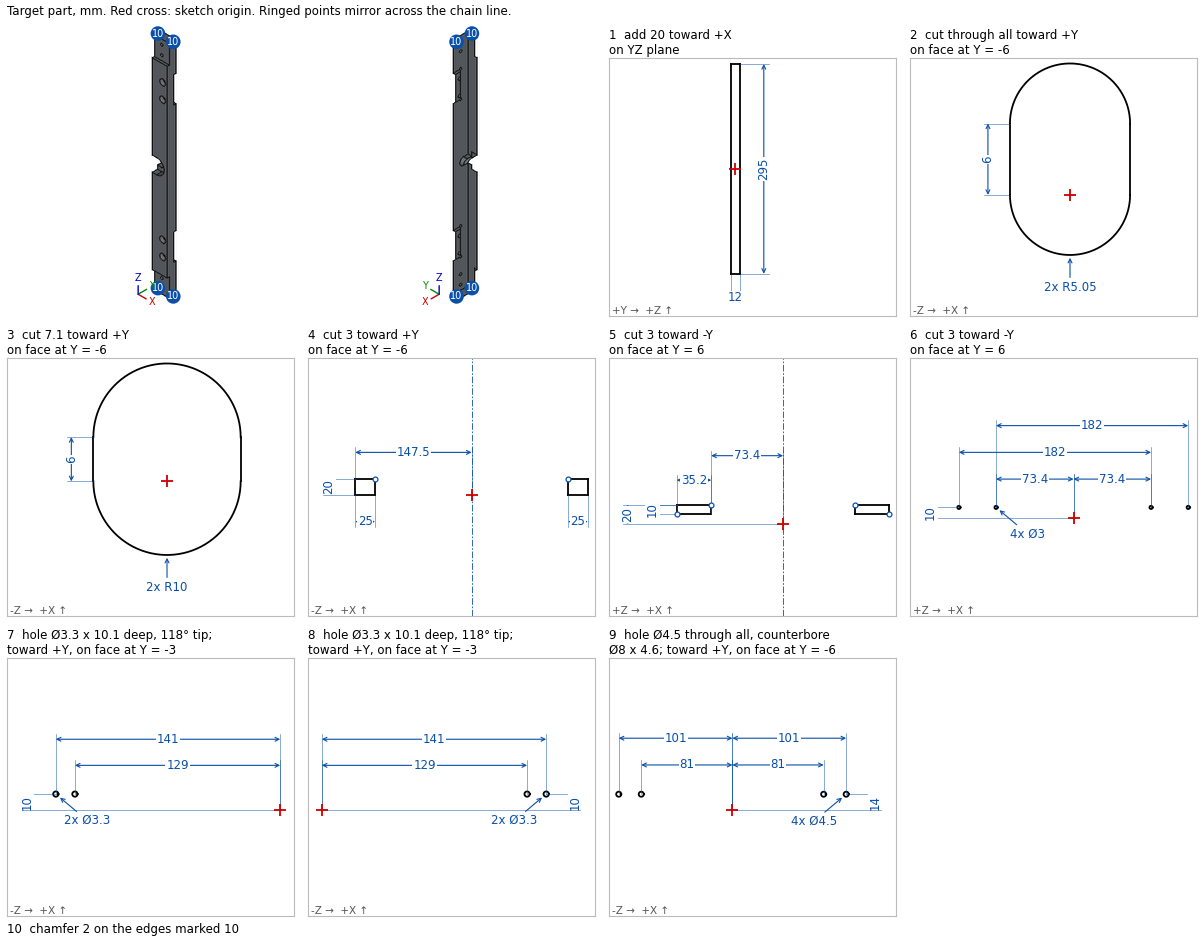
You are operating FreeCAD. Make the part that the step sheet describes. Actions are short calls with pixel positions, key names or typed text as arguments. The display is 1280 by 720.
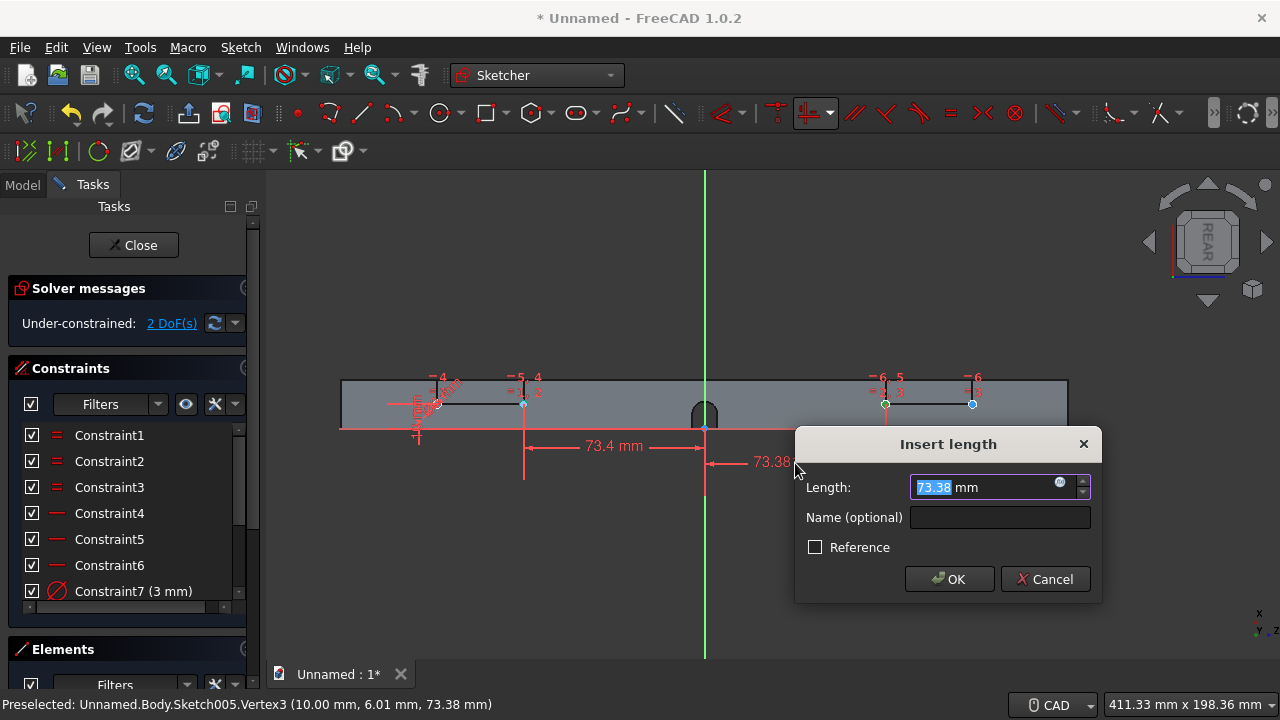
text(73.4)
key(Return)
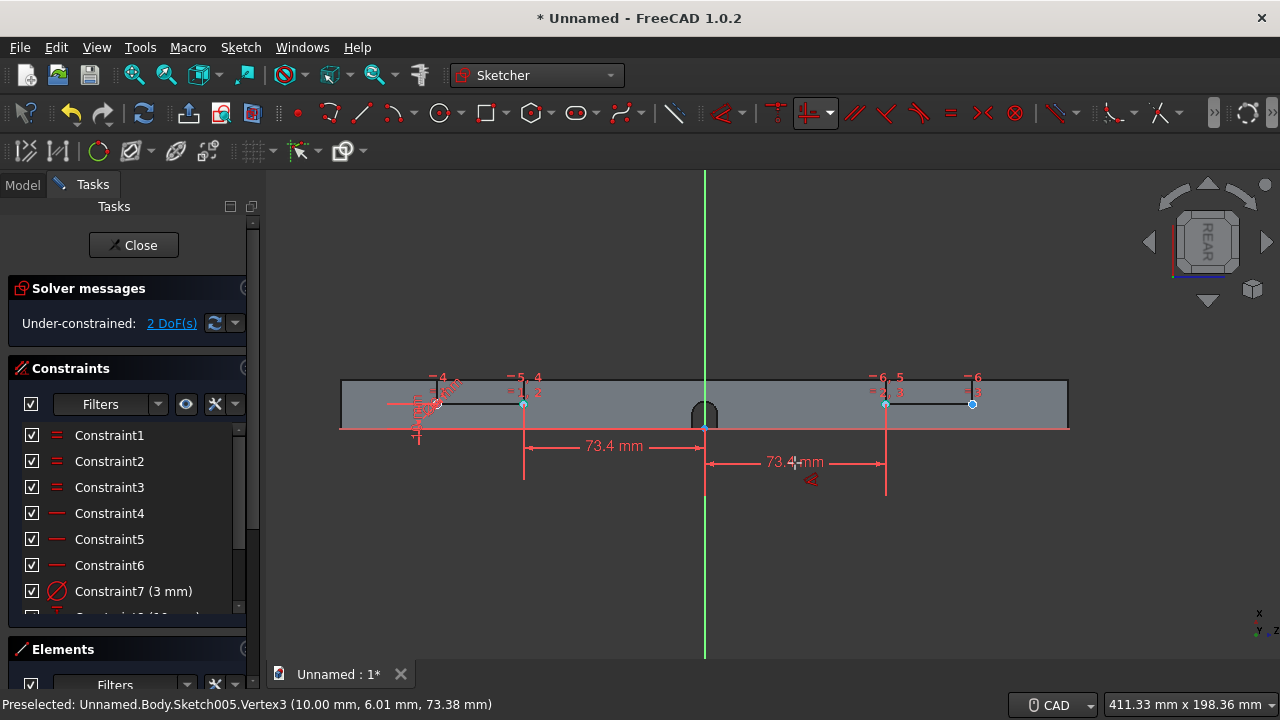
click(437, 404)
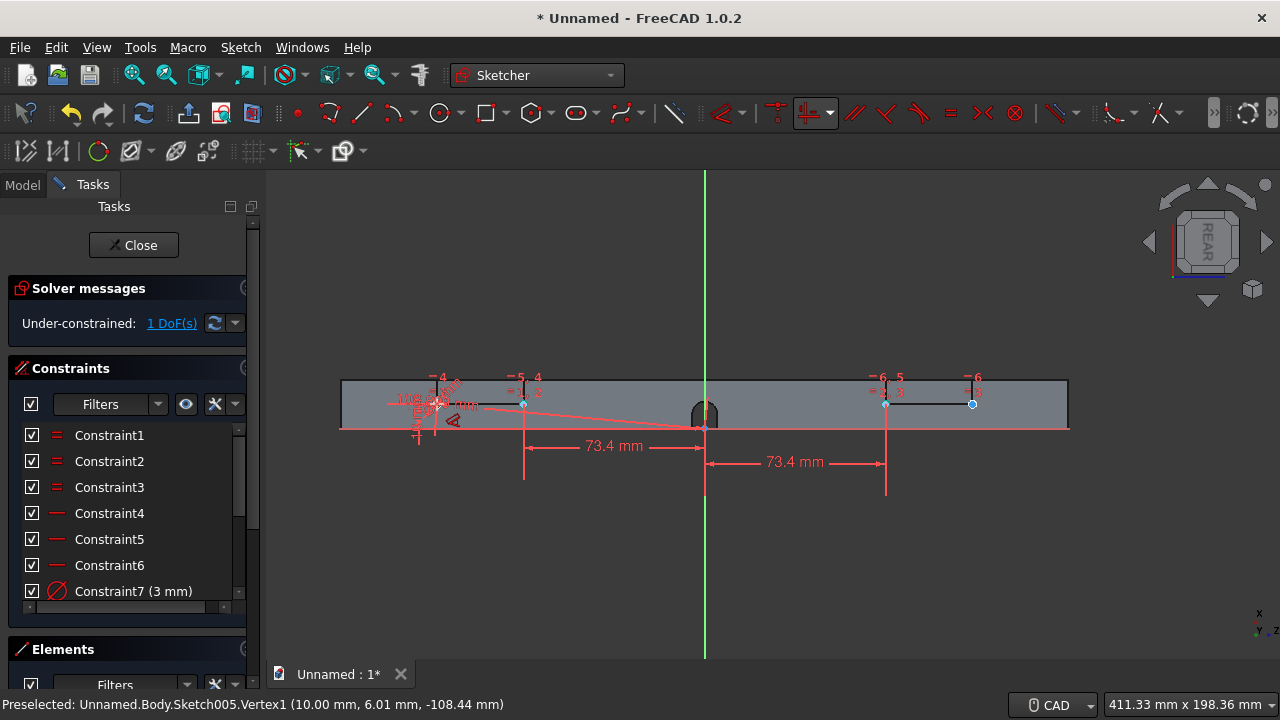
click(886, 404)
click(662, 370)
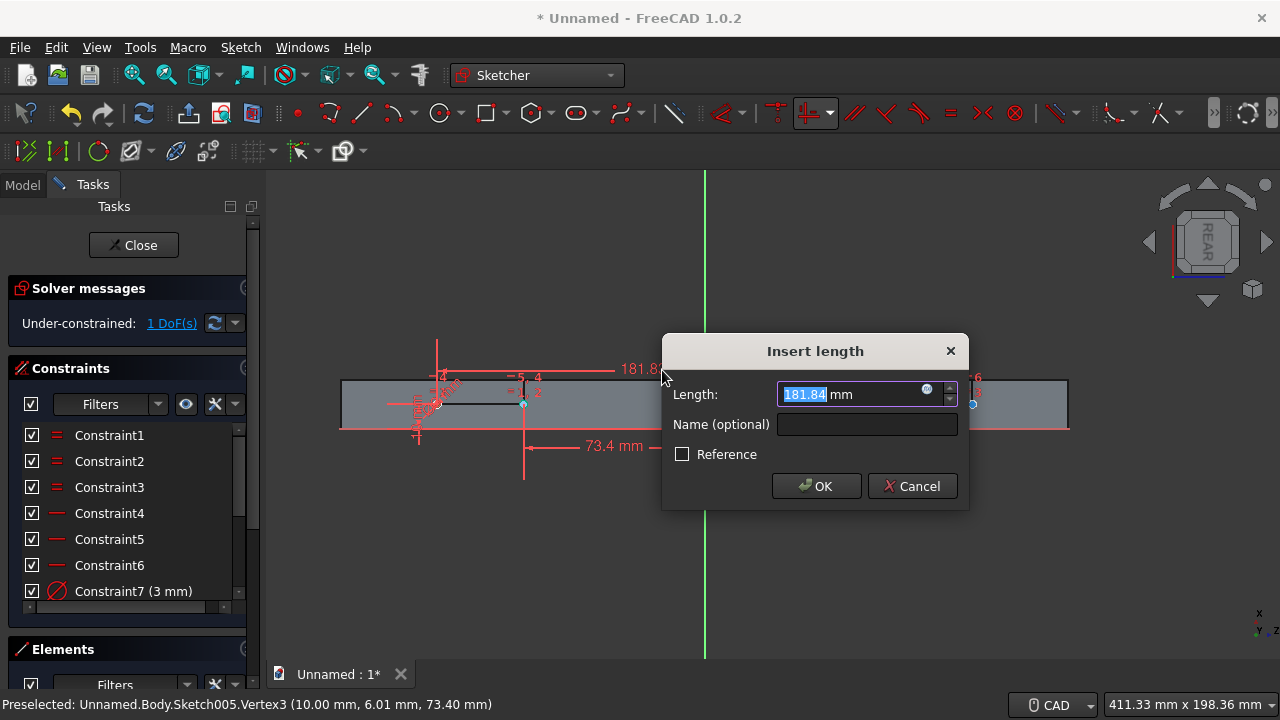
text(182)
key(Return)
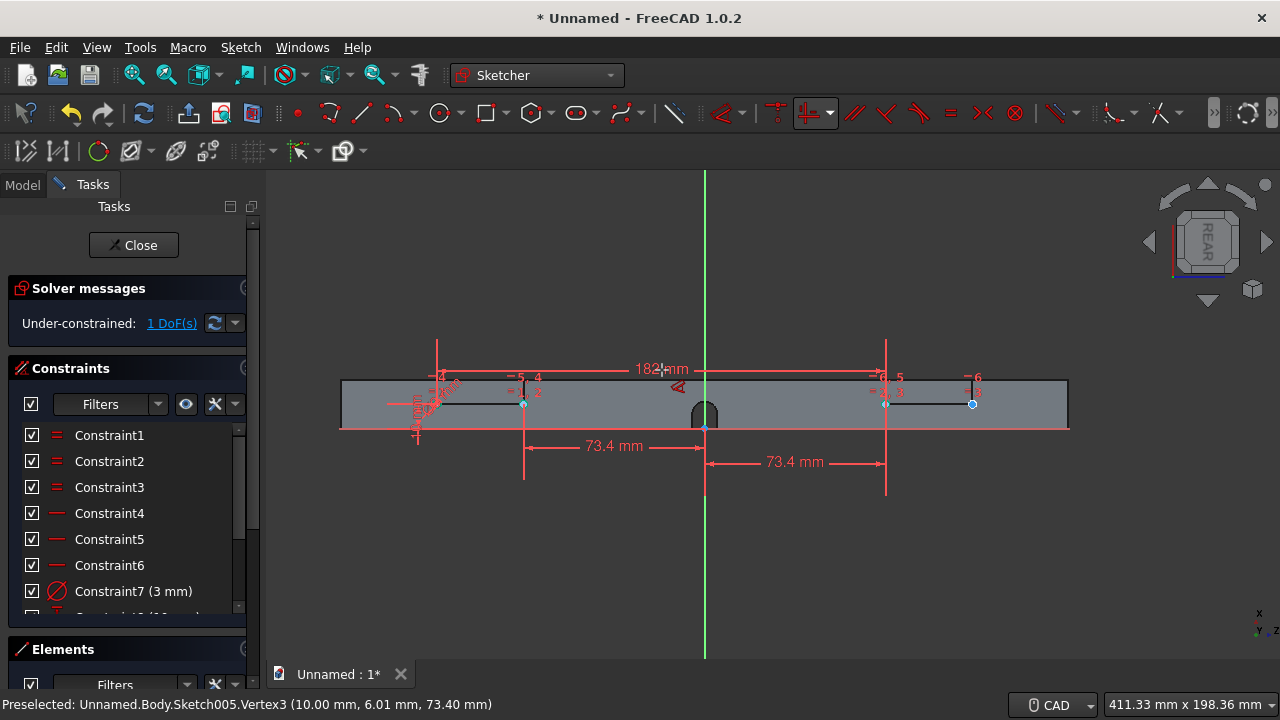
click(524, 404)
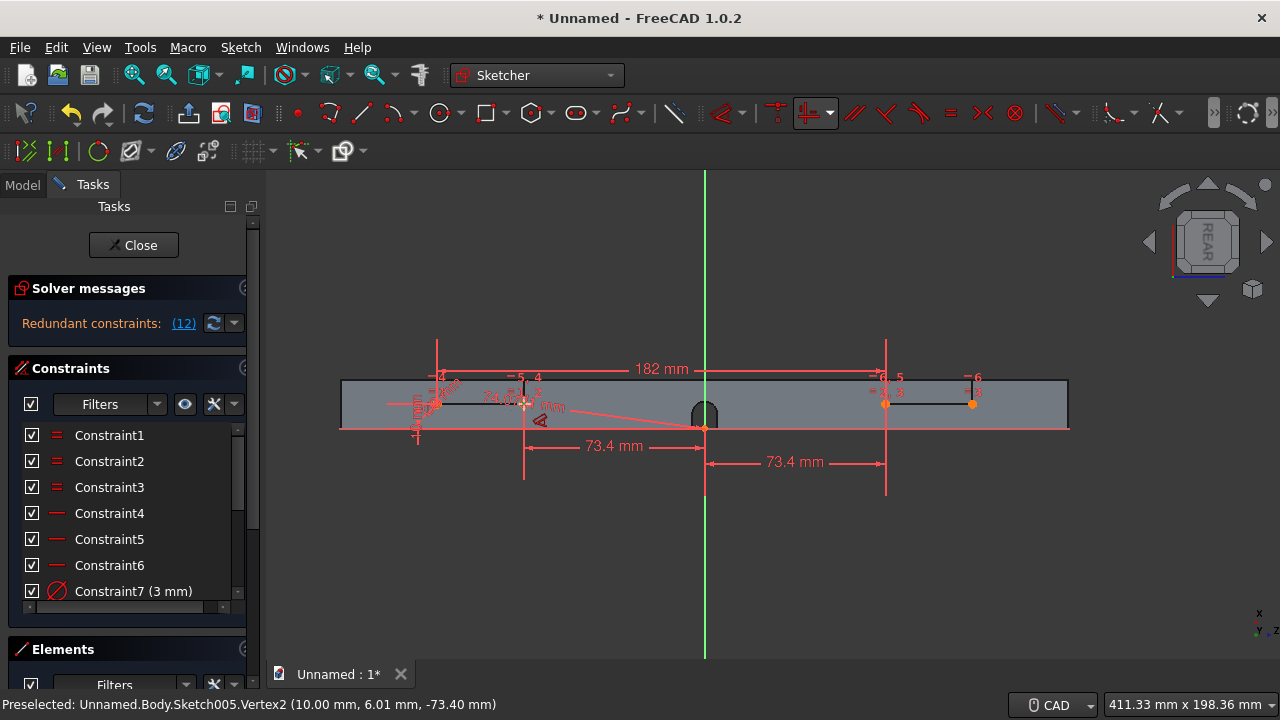
click(973, 404)
click(748, 370)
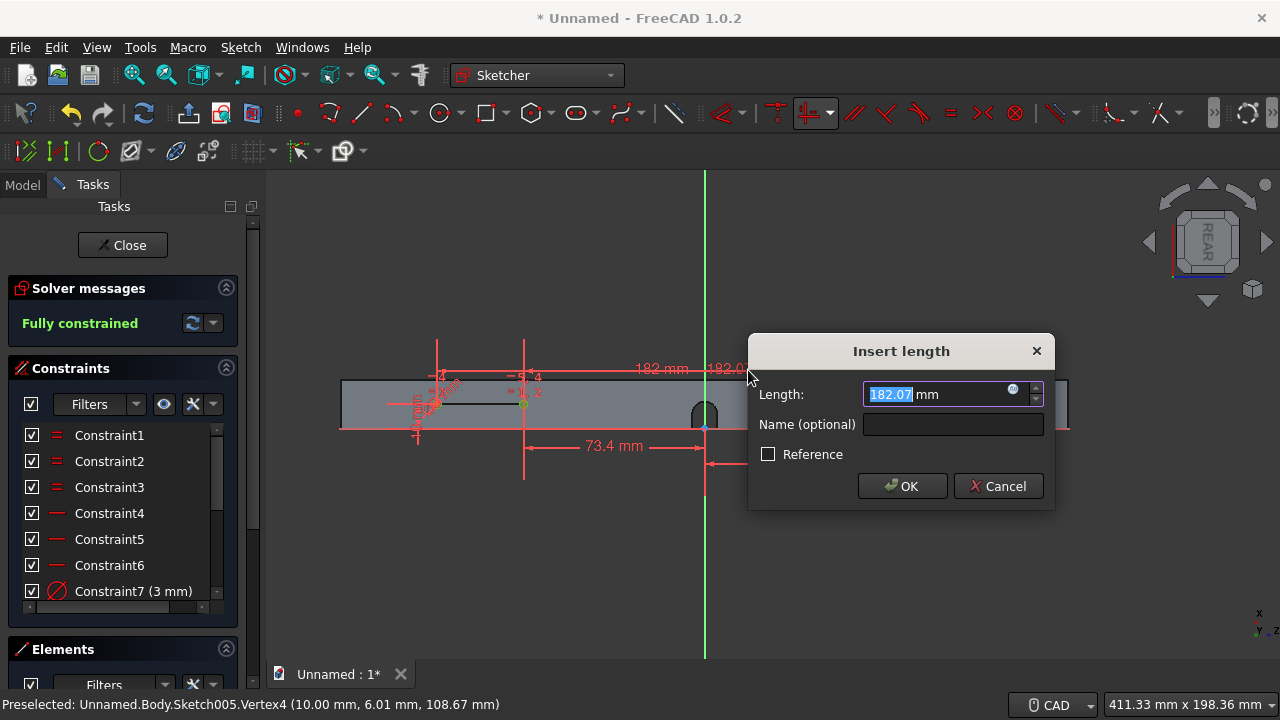
text(182)
key(Return)
key(Escape)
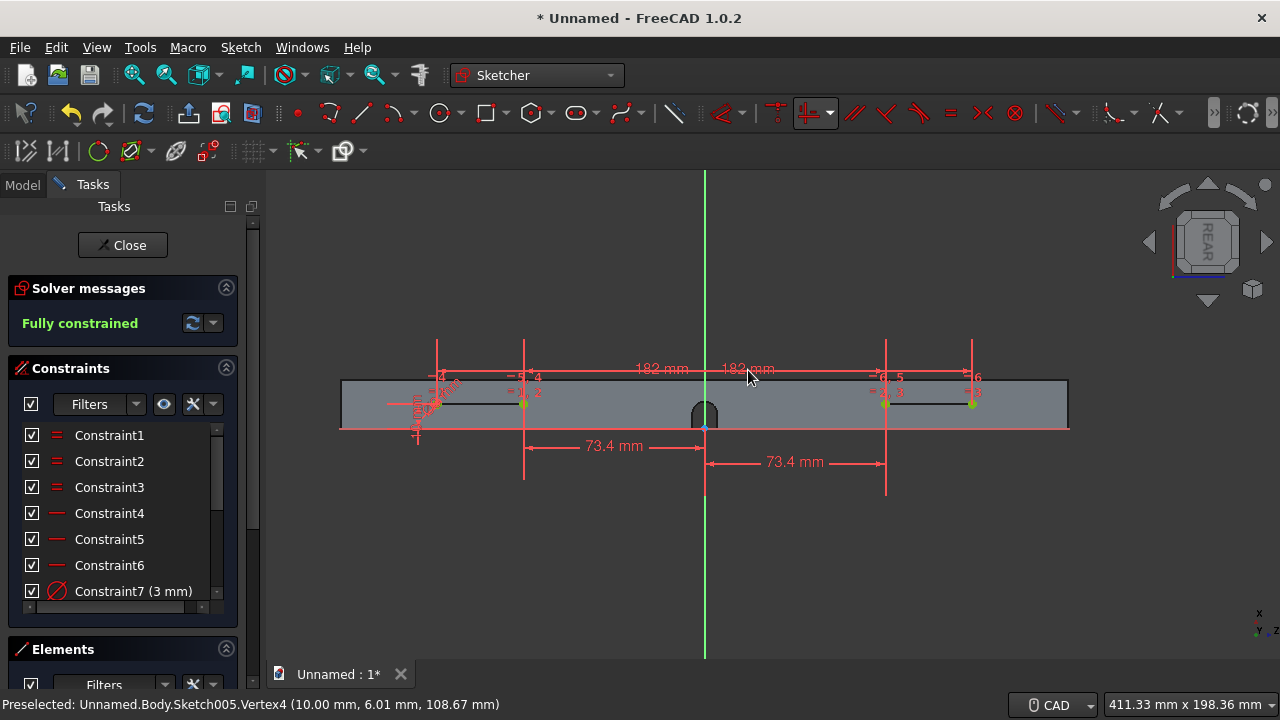
click(123, 245)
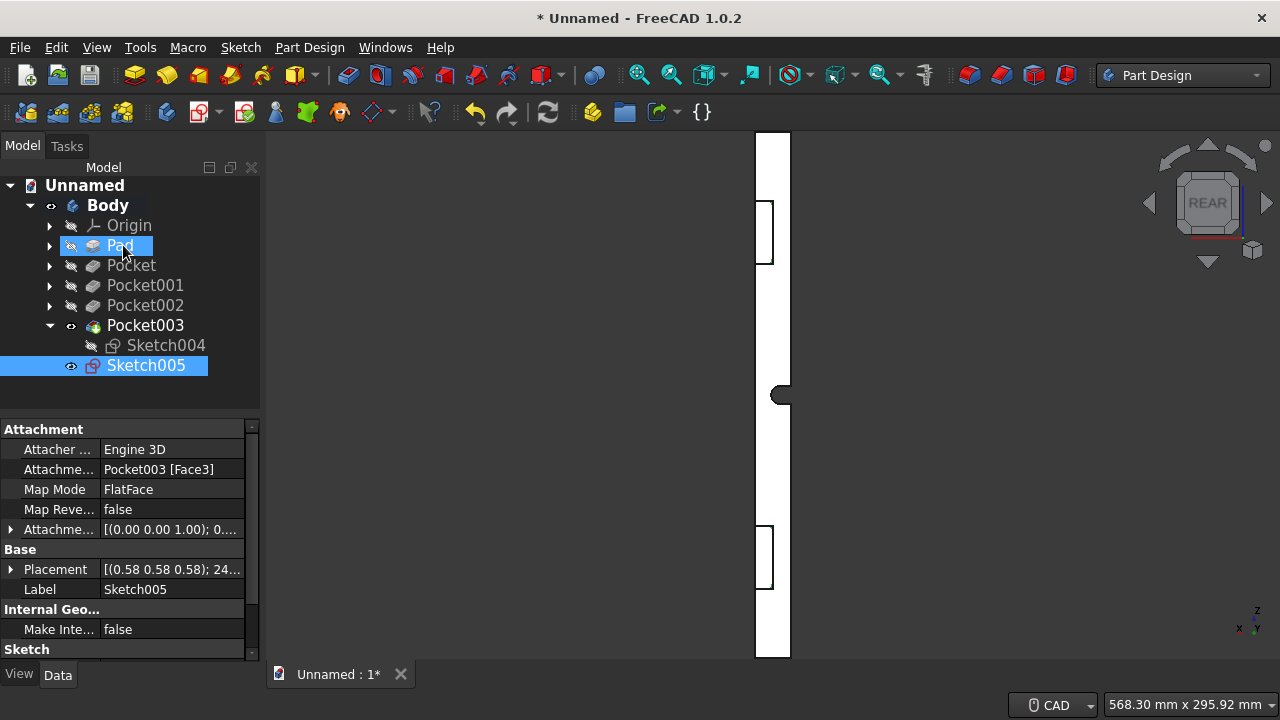
click(350, 76)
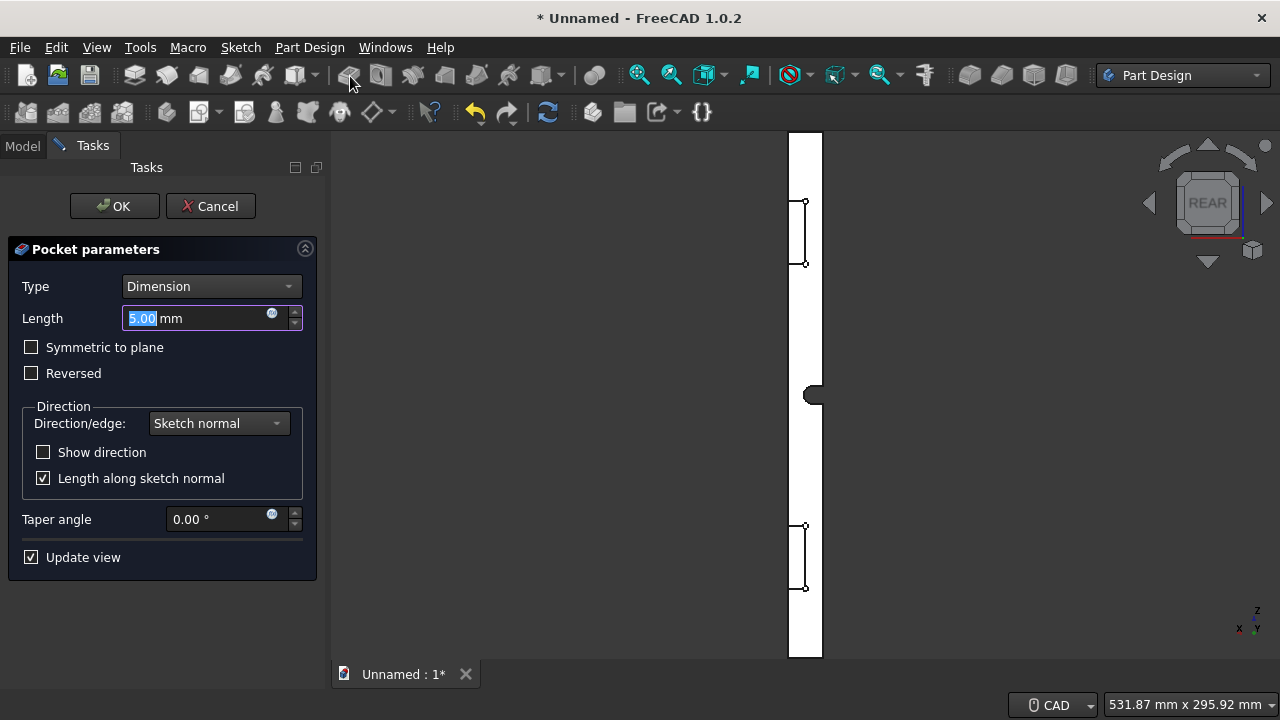
text(3)
key(Tab)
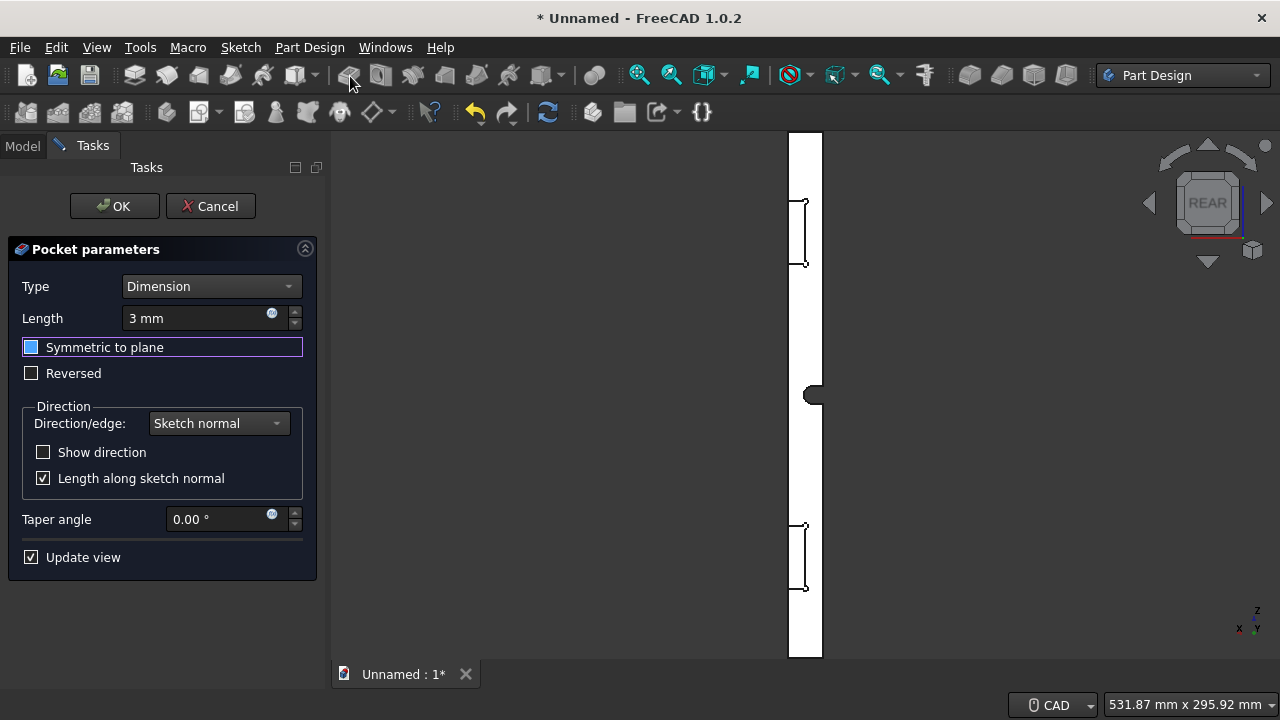
click(115, 206)